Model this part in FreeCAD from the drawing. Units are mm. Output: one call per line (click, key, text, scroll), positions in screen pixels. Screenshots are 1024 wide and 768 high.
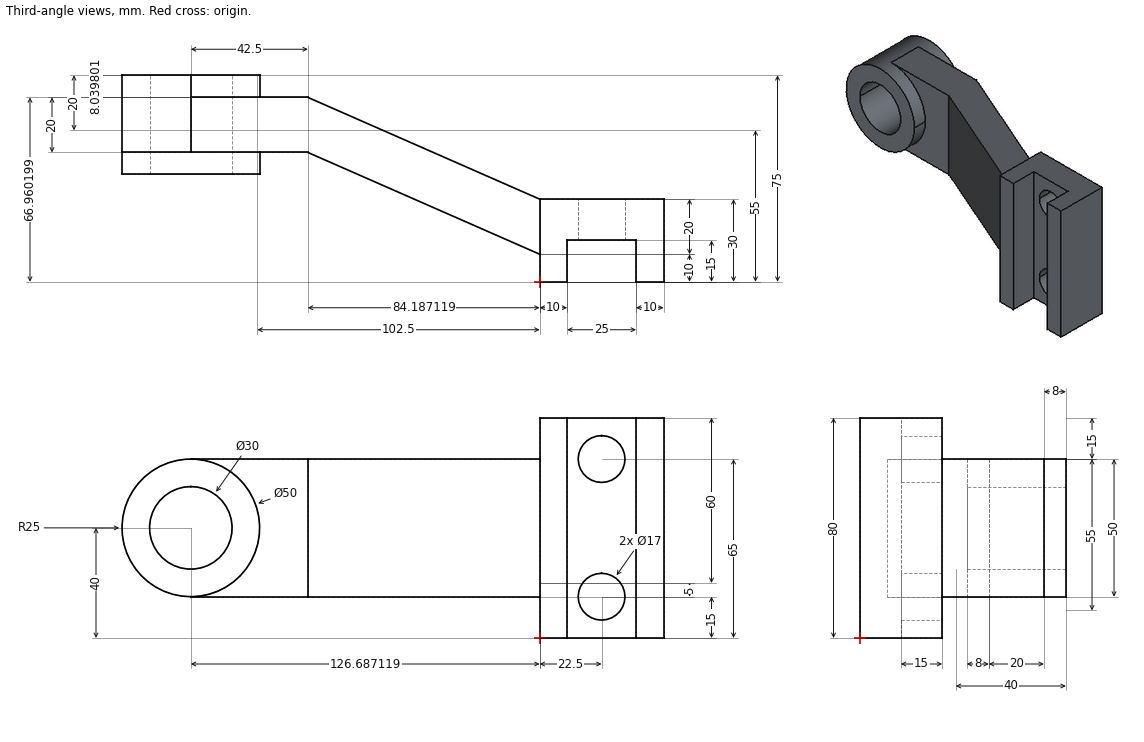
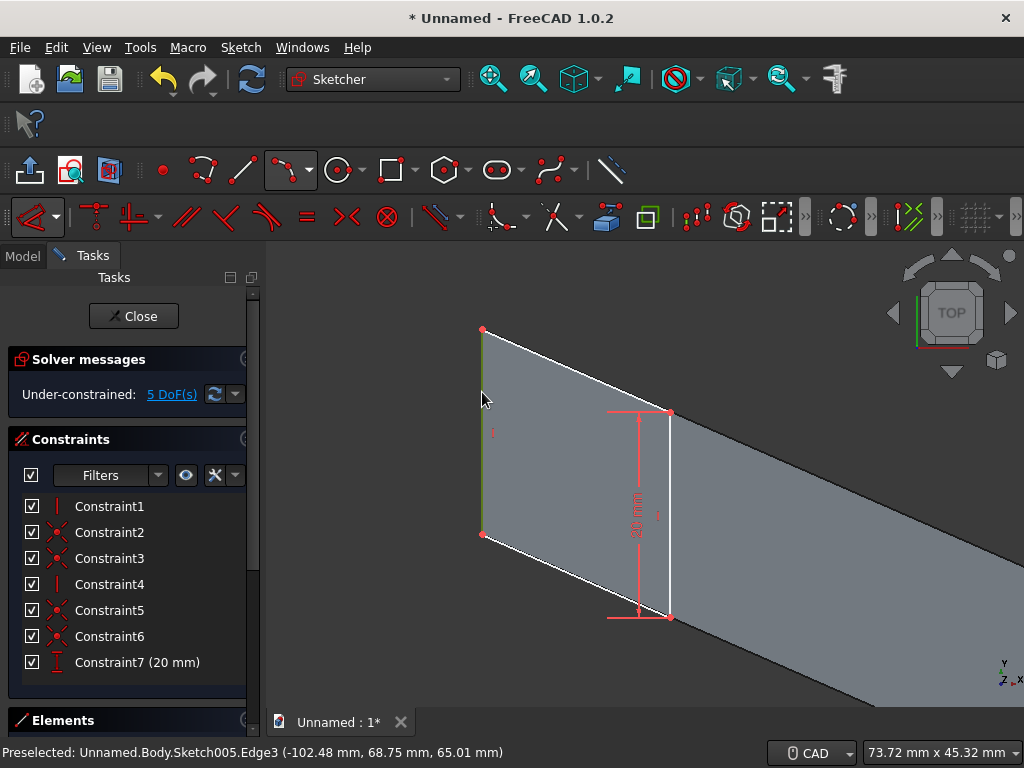
key(i)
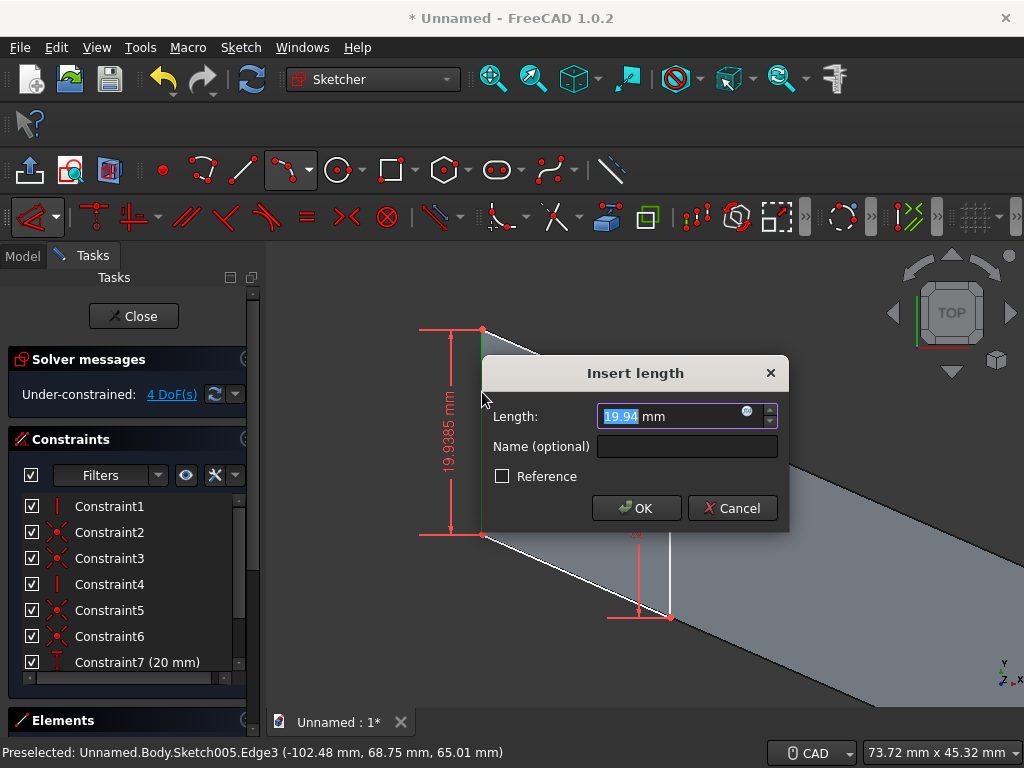
text(20)
key(Return)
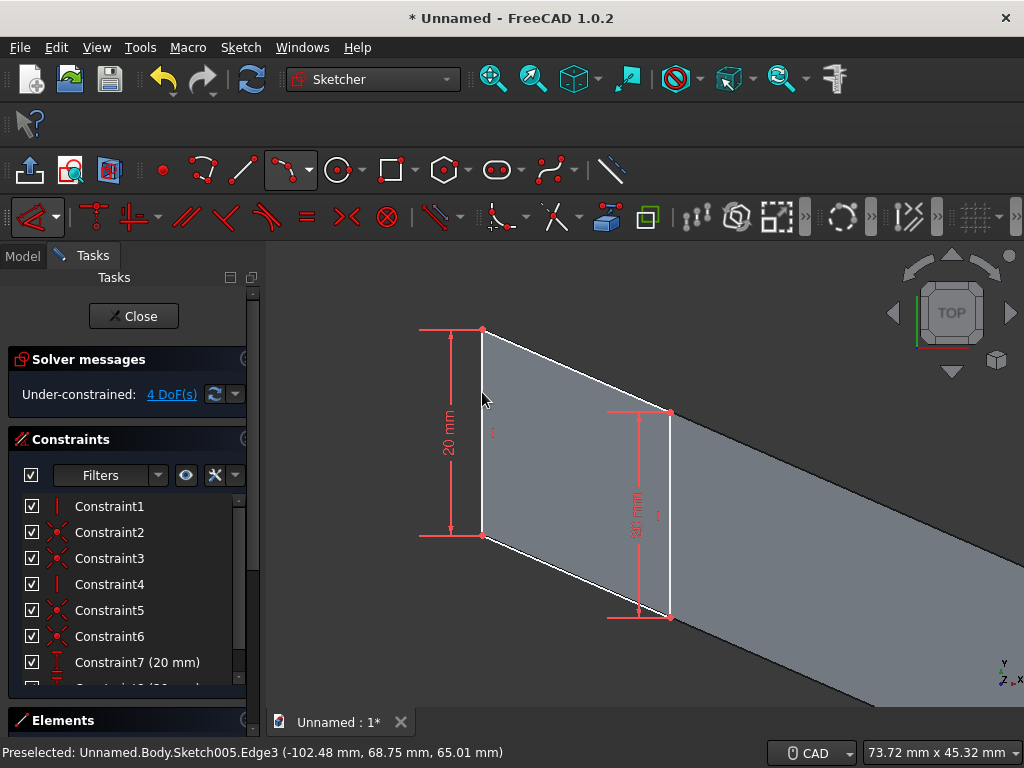
click(482, 330)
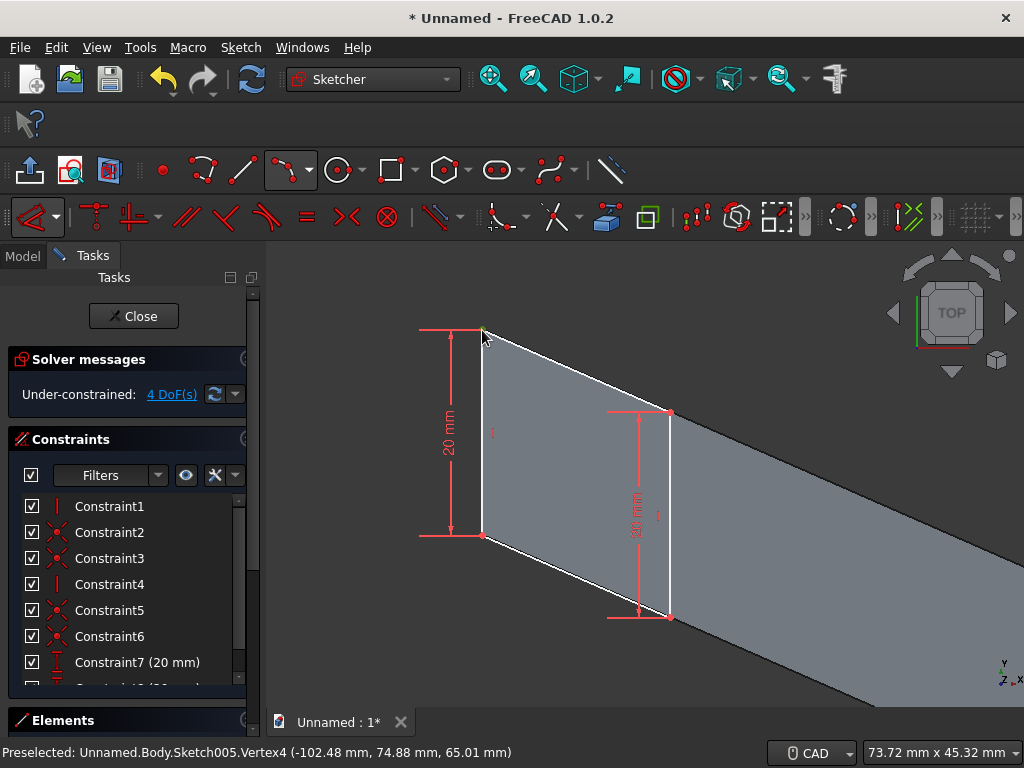
key(i)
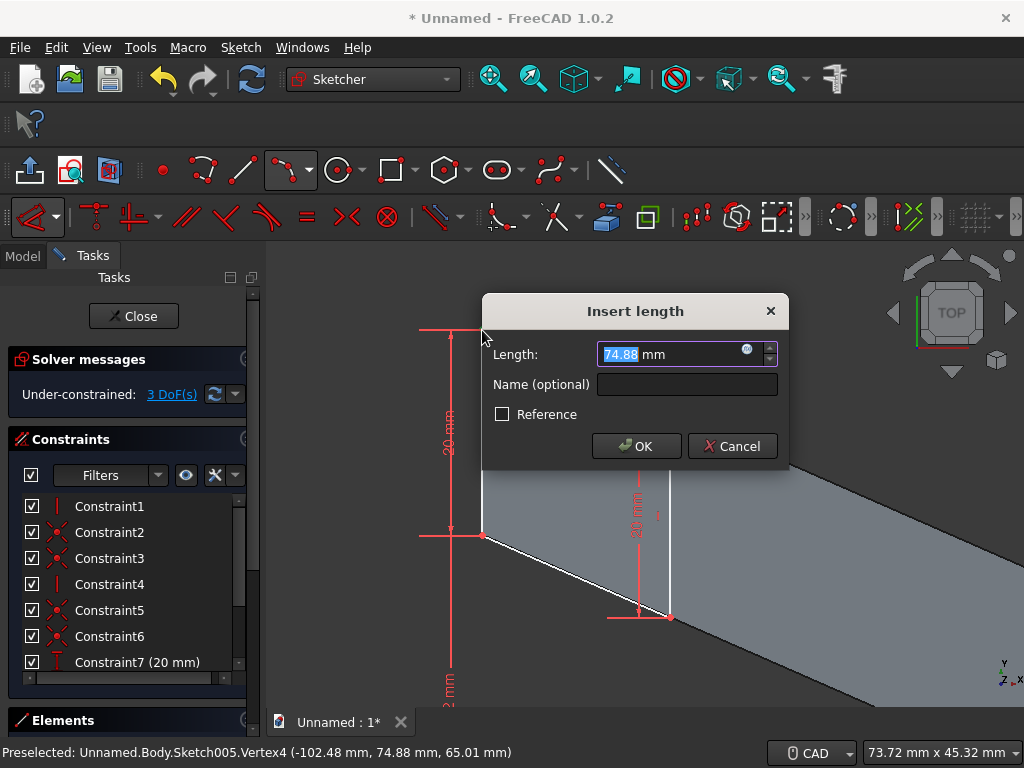
text(75)
key(Return)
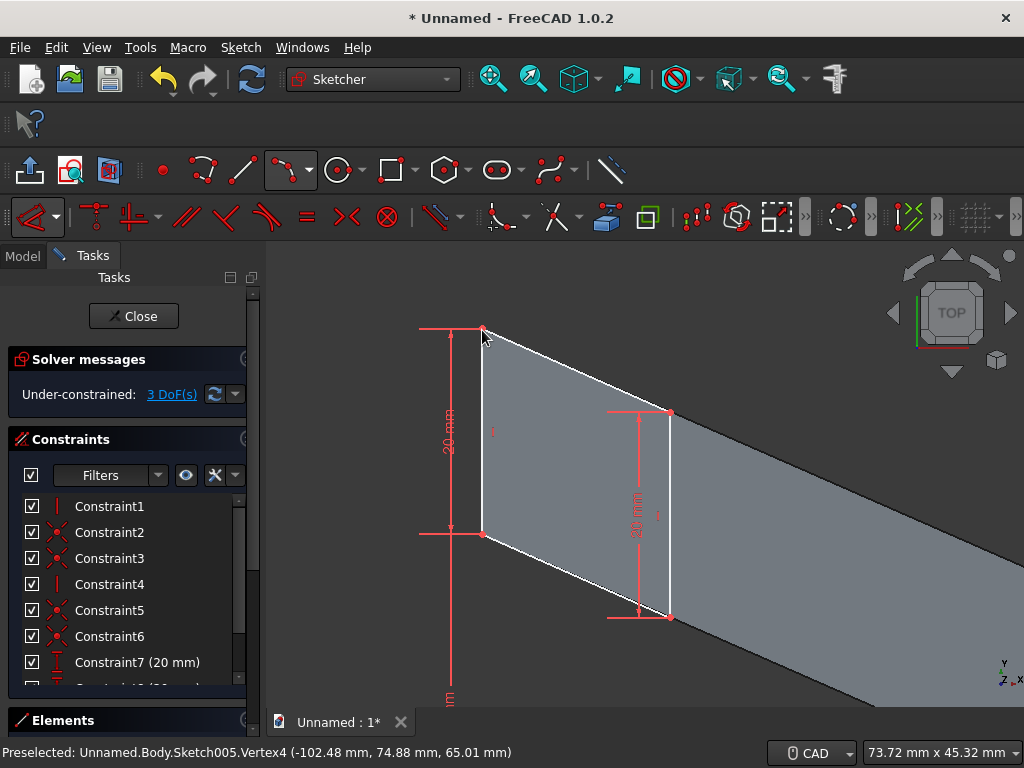
click(482, 329)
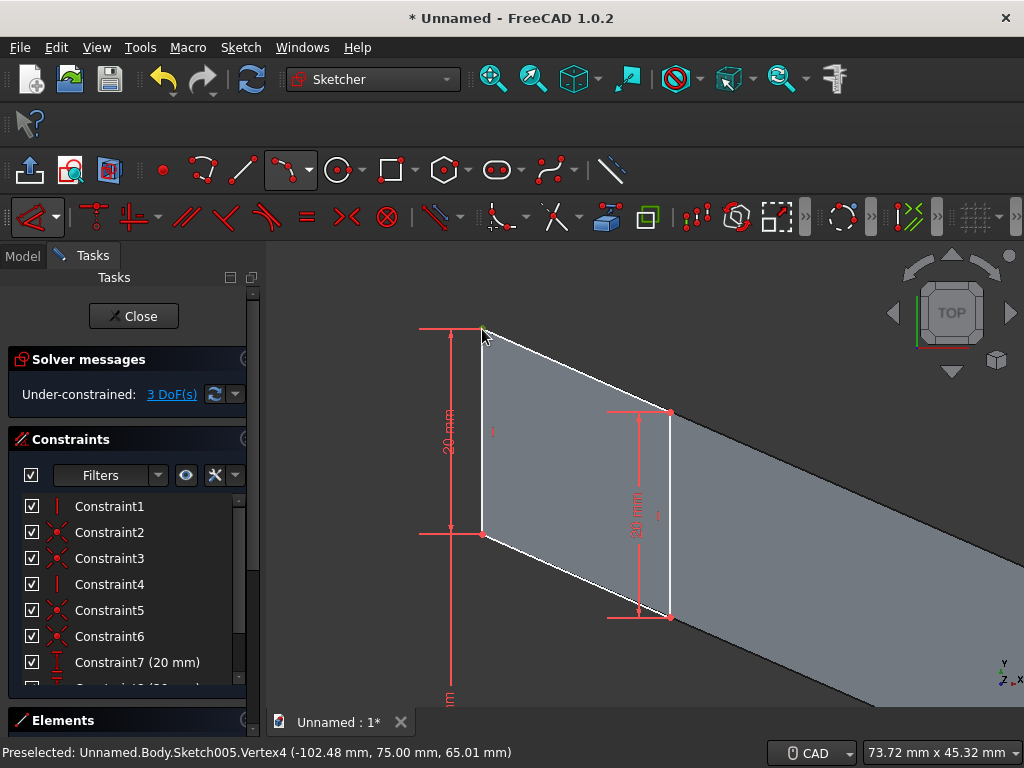
key(l)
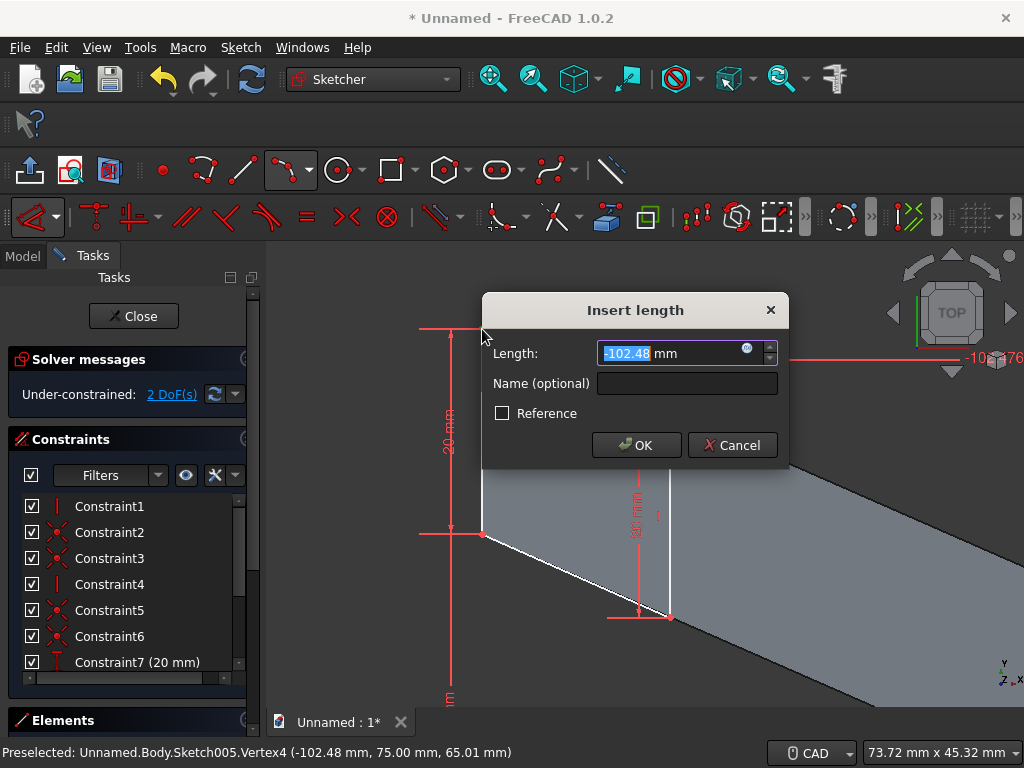
text(-102.5)
key(Return)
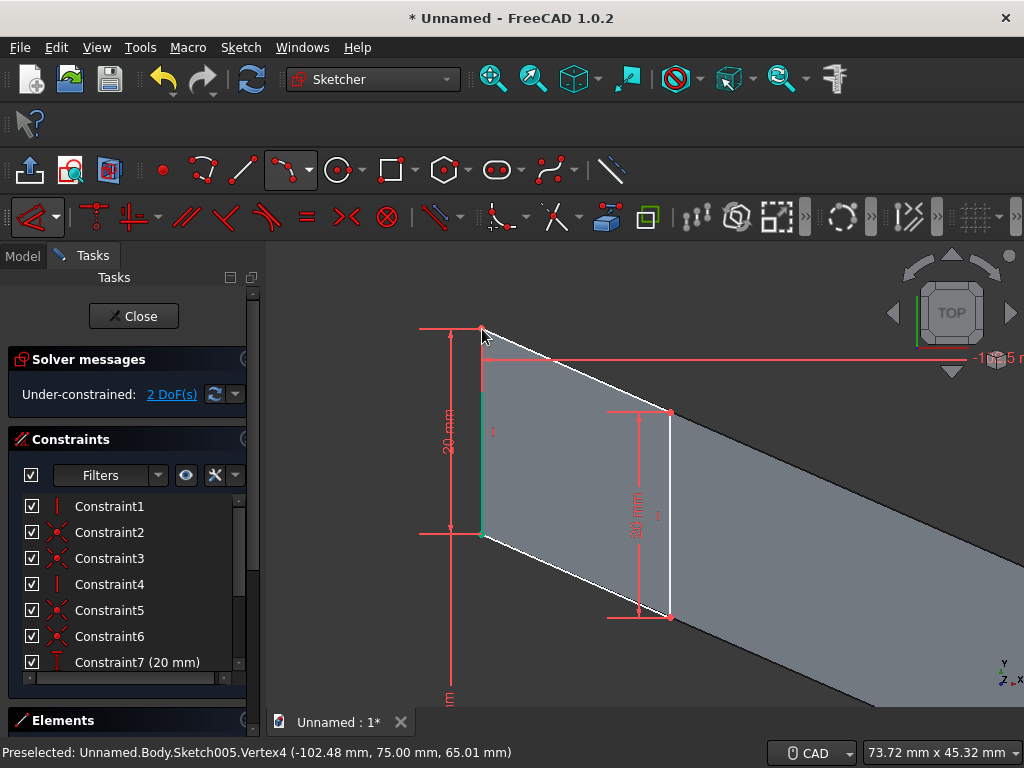
click(614, 387)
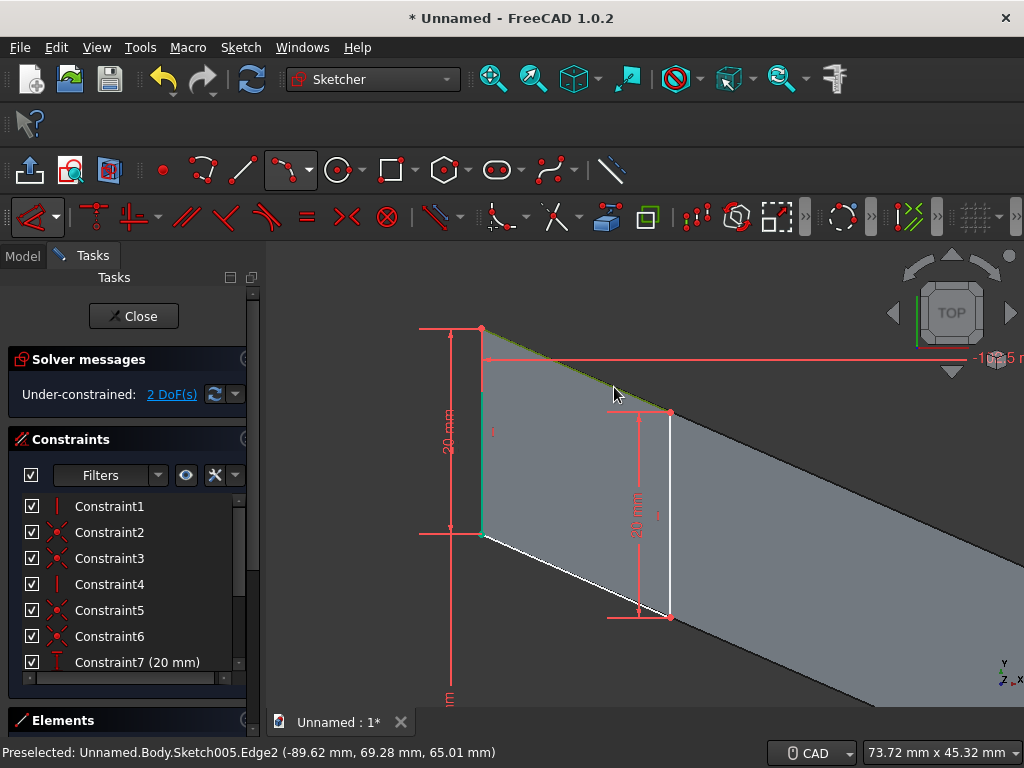
key(i)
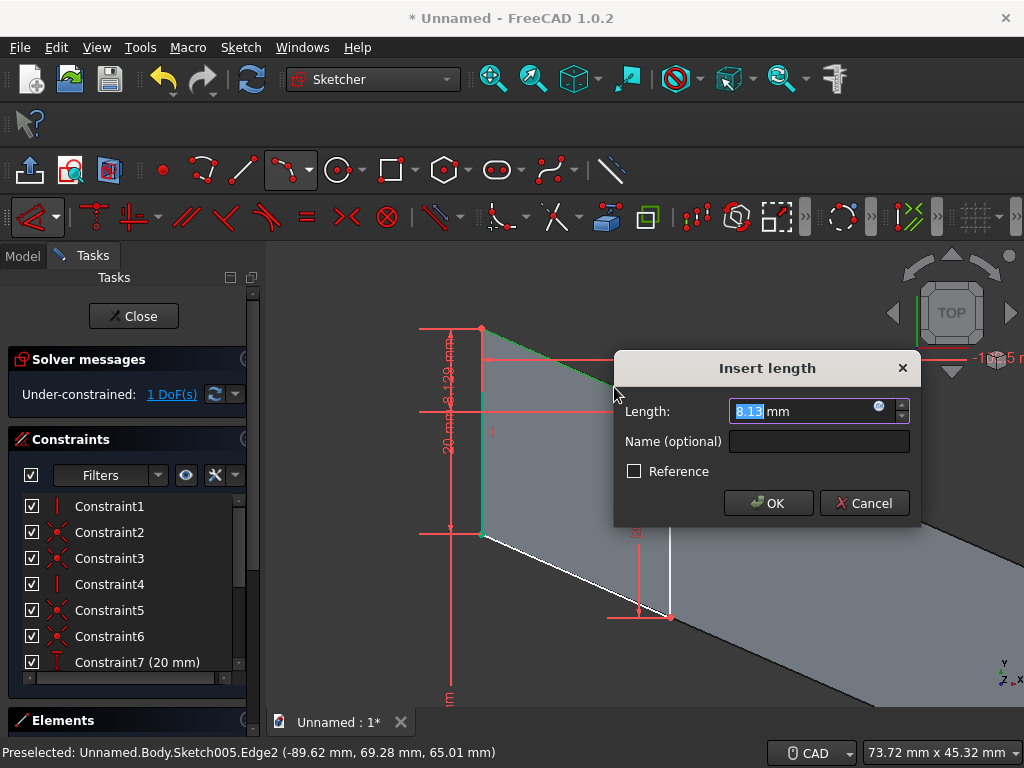
text(8.039801)
key(Return)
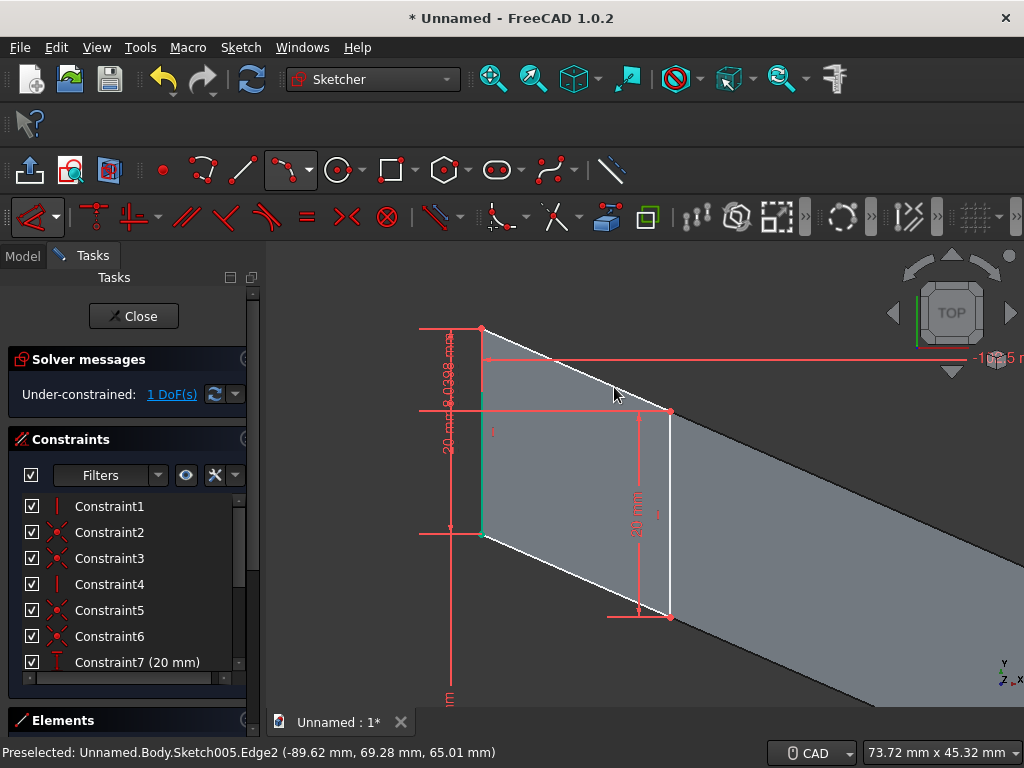
click(670, 617)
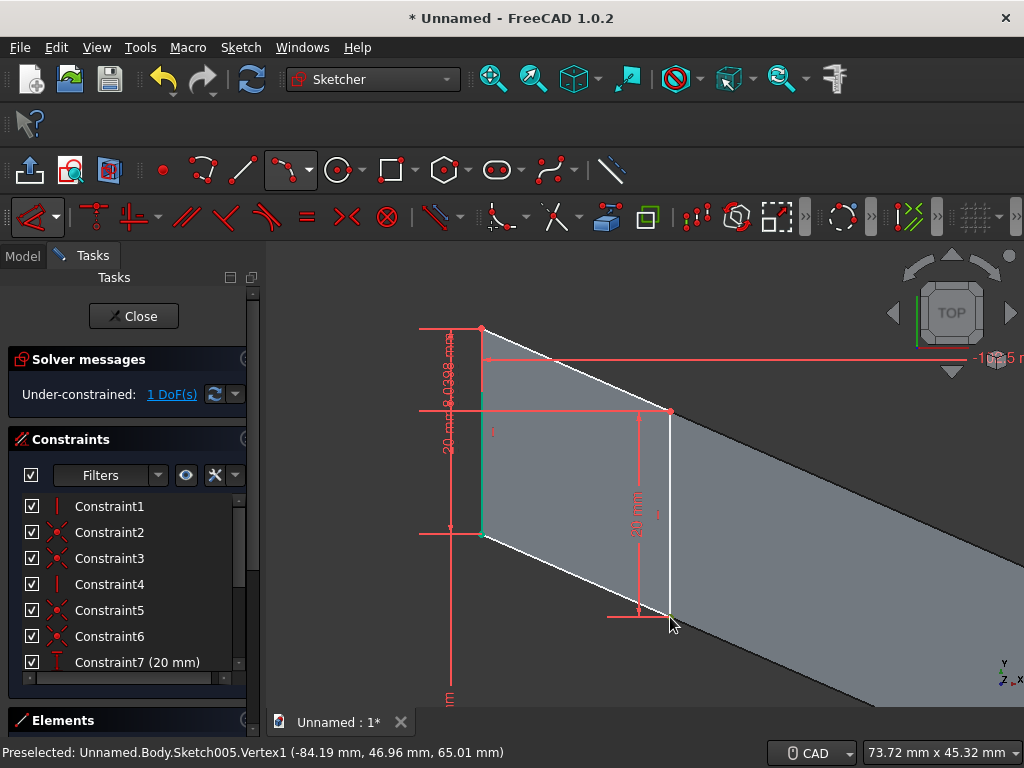
key(l)